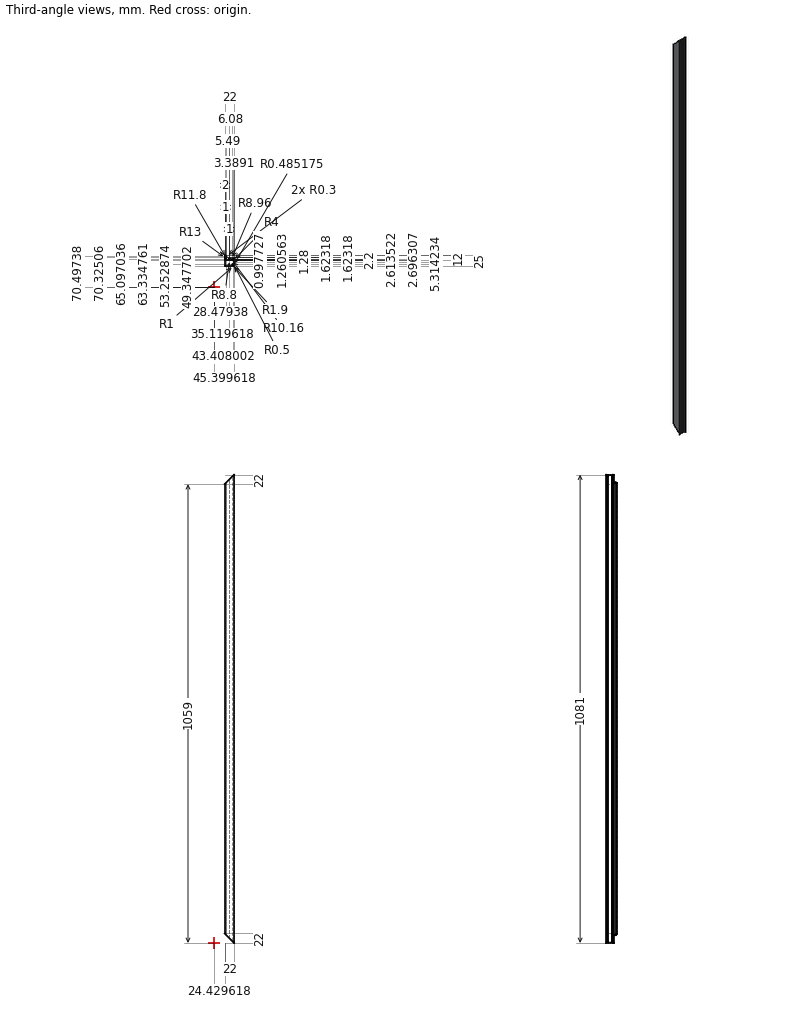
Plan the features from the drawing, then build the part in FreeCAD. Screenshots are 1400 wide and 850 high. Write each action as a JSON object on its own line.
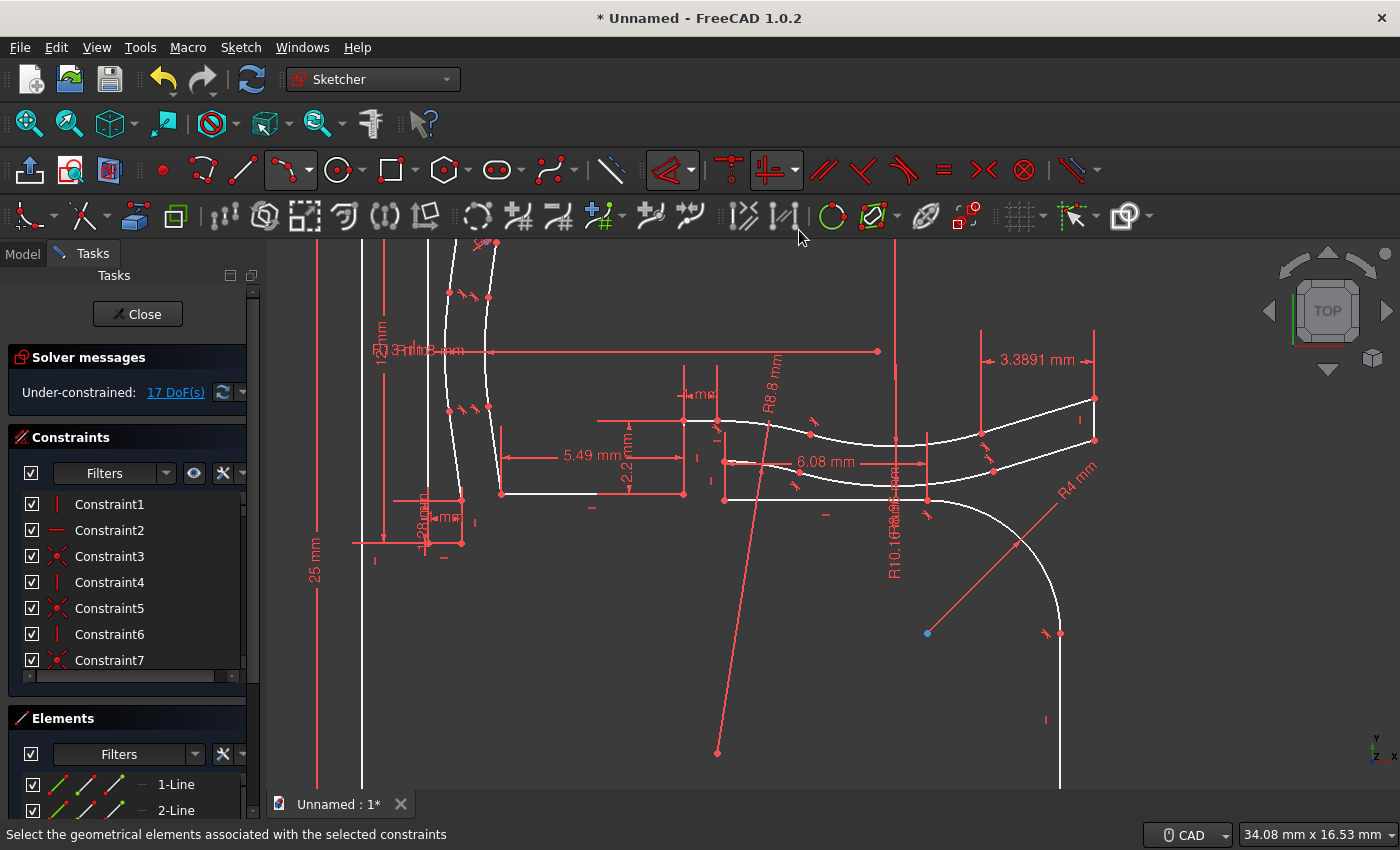
{"action": "left_click", "coordinate": [1060, 753]}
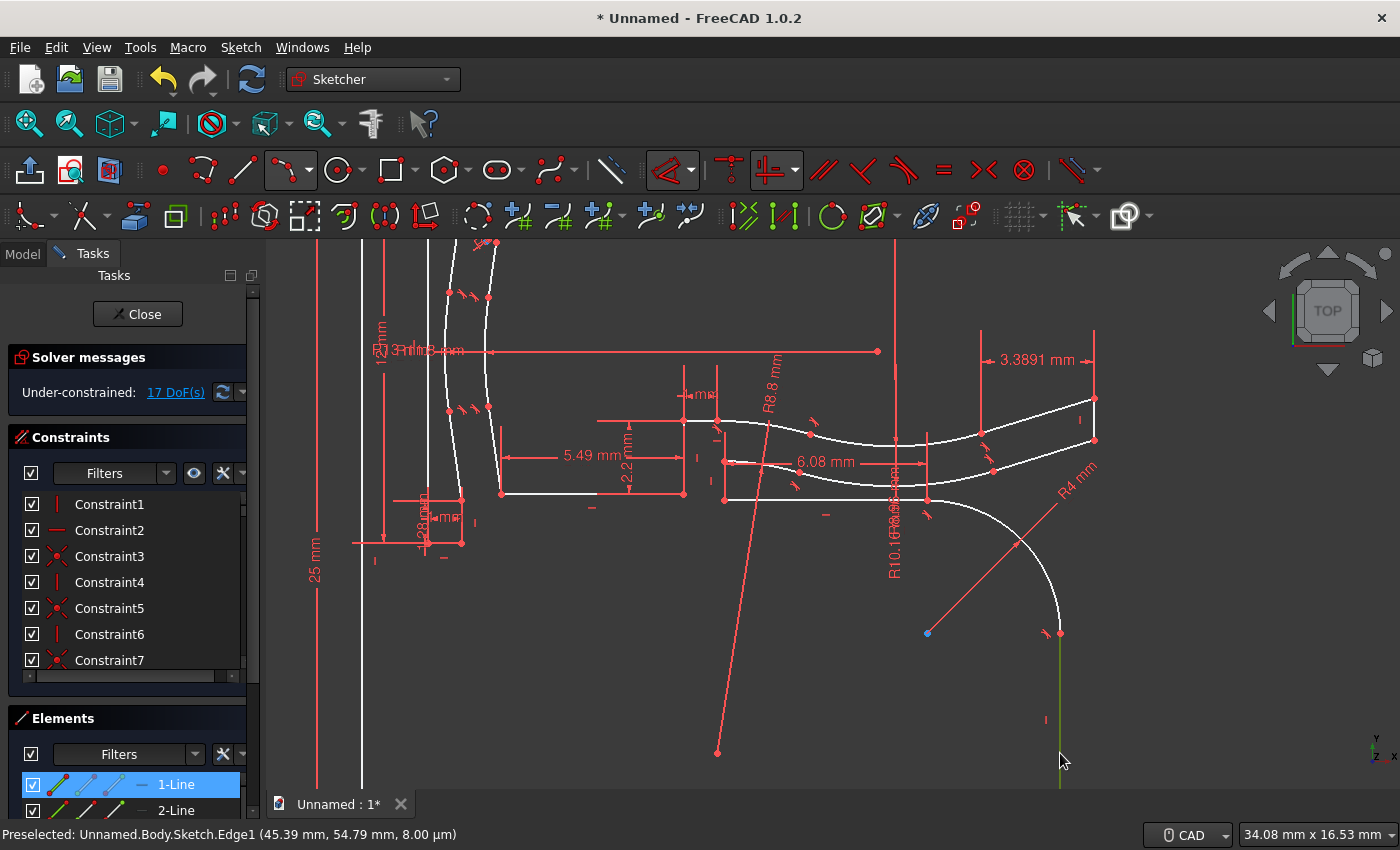
{"action": "left_click", "coordinate": [694, 170]}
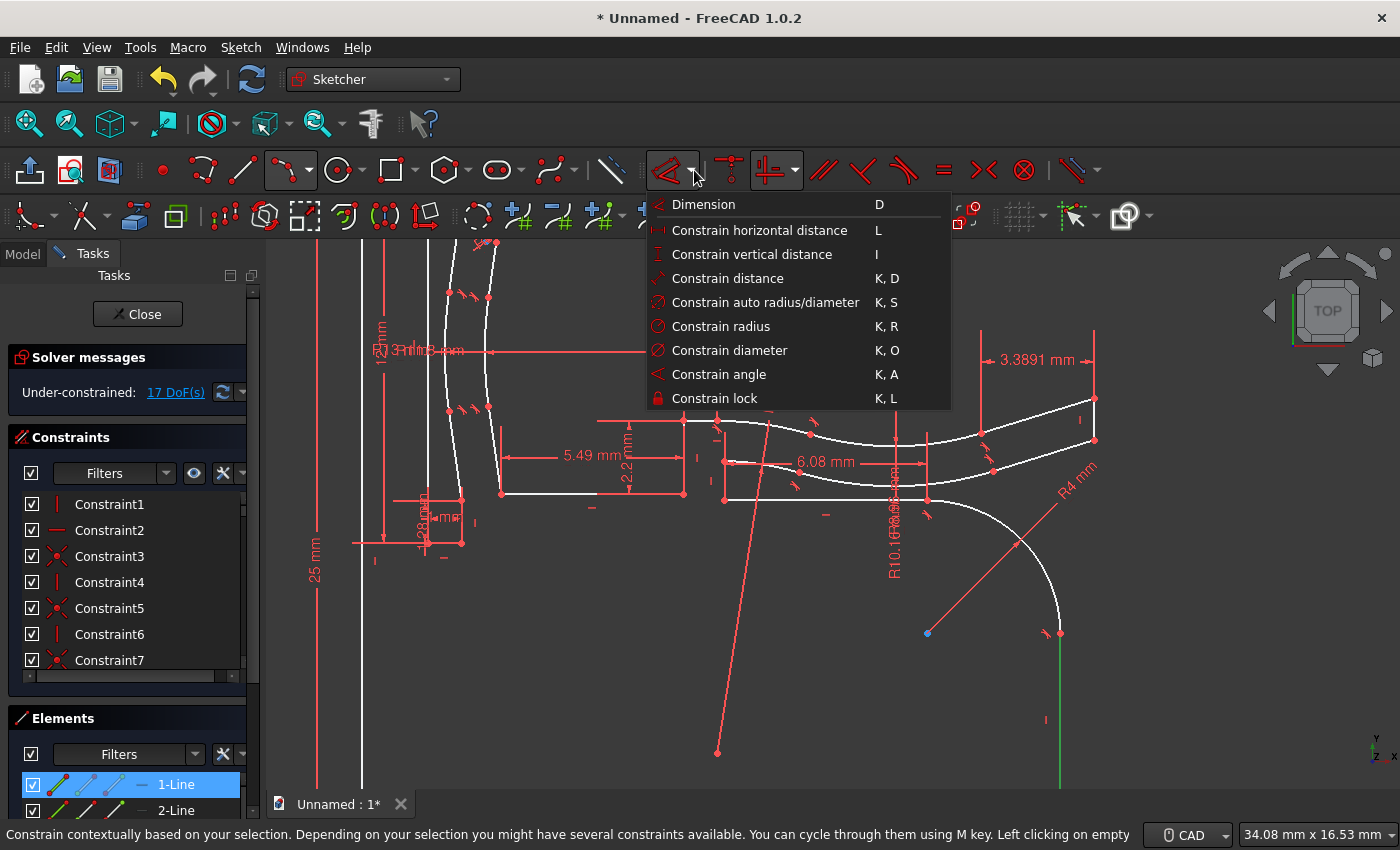
{"action": "left_click", "coordinate": [799, 254]}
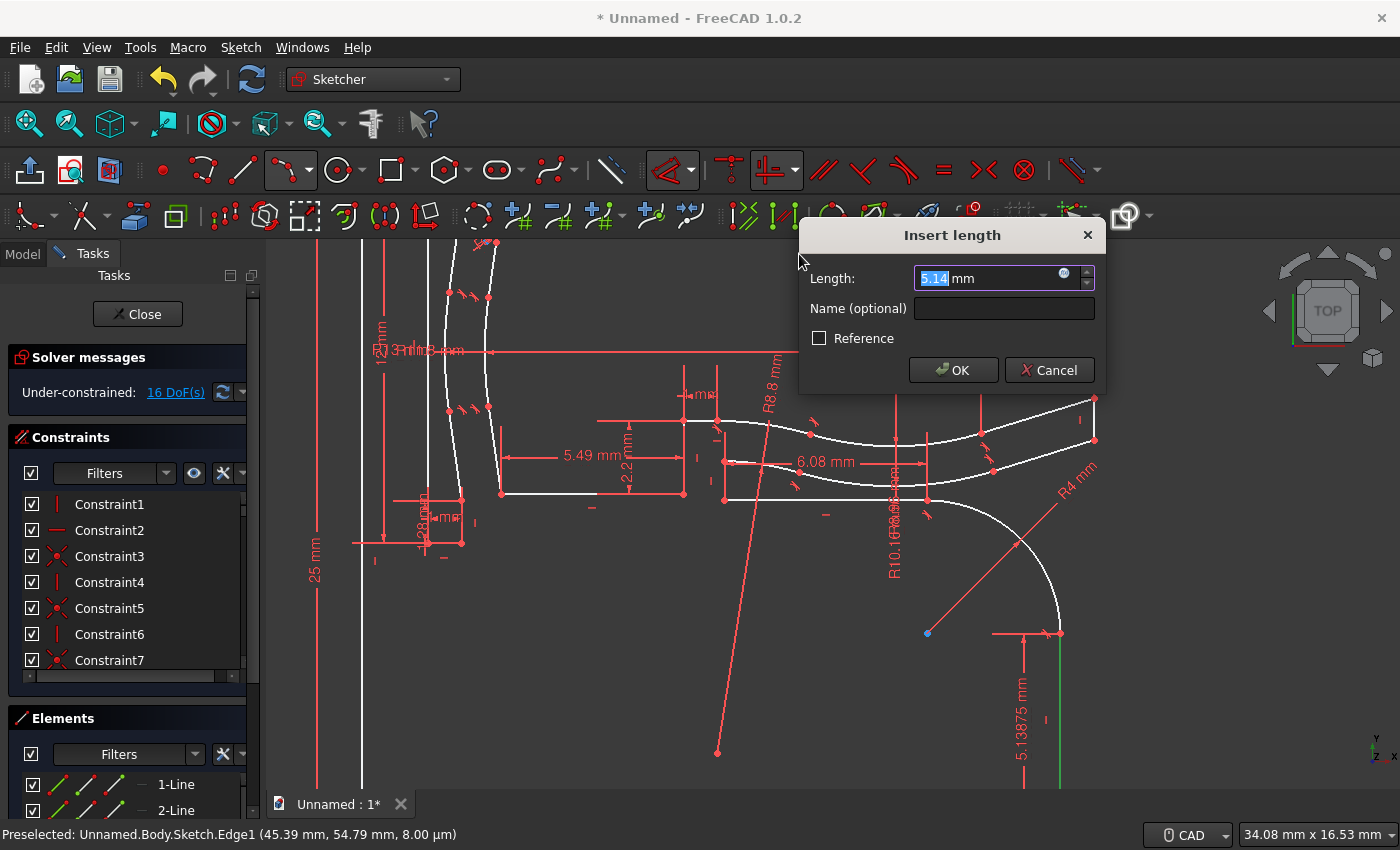
{"action": "type", "text": "5.314234"}
{"action": "key", "text": "Return"}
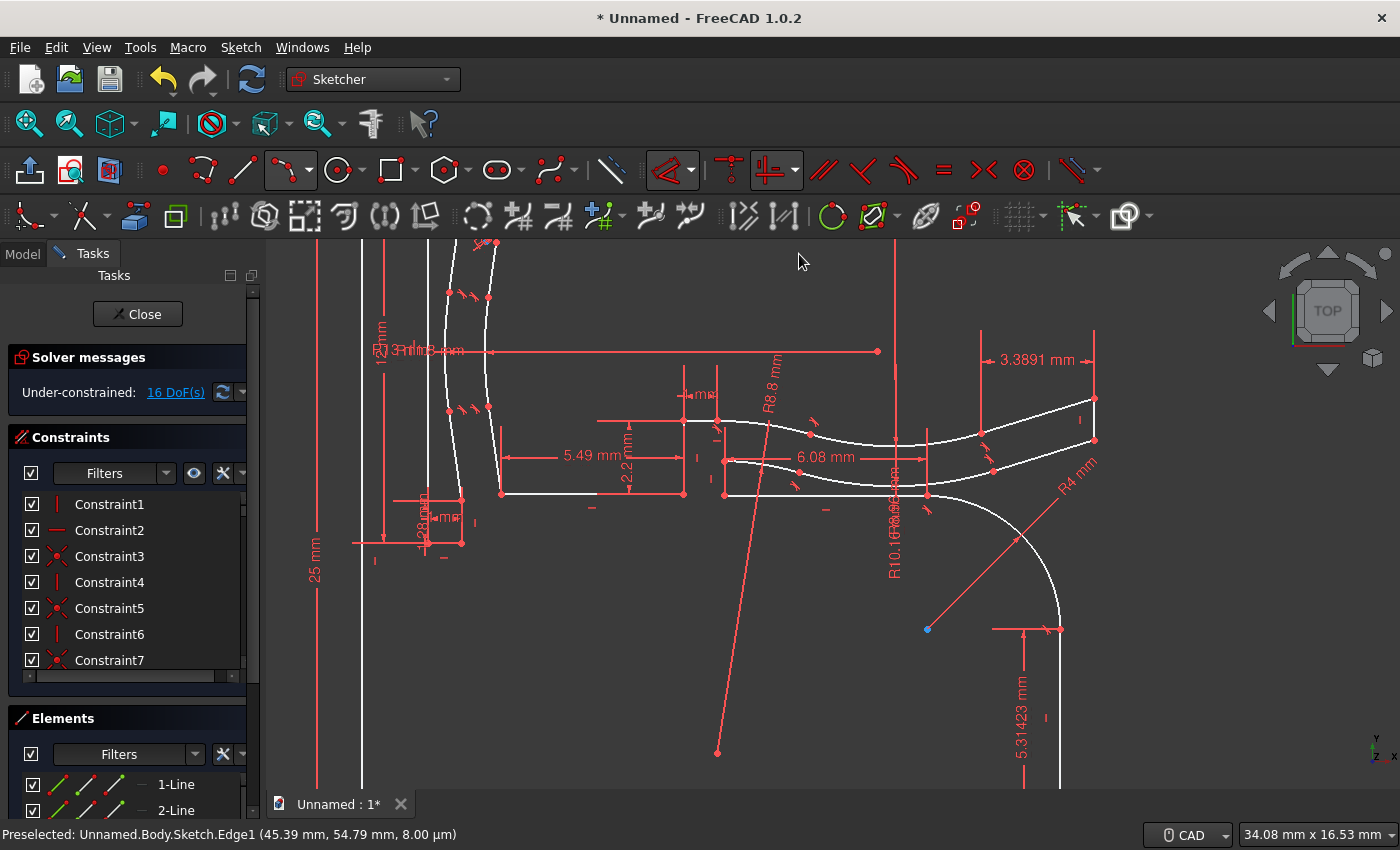
{"action": "scroll", "coordinate": [725, 485], "scroll_direction": "up", "scroll_amount": 2}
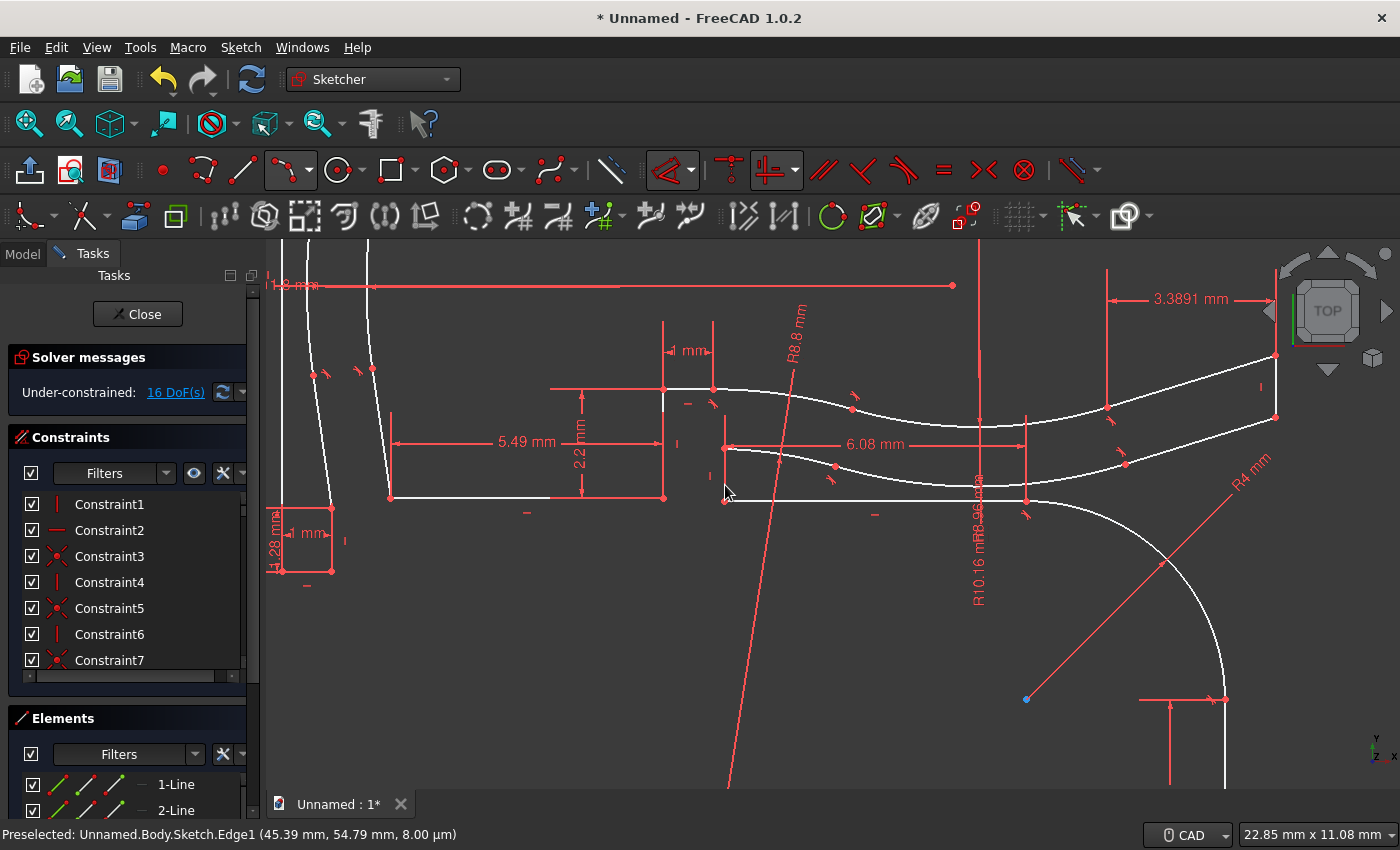
{"action": "left_click", "coordinate": [725, 485]}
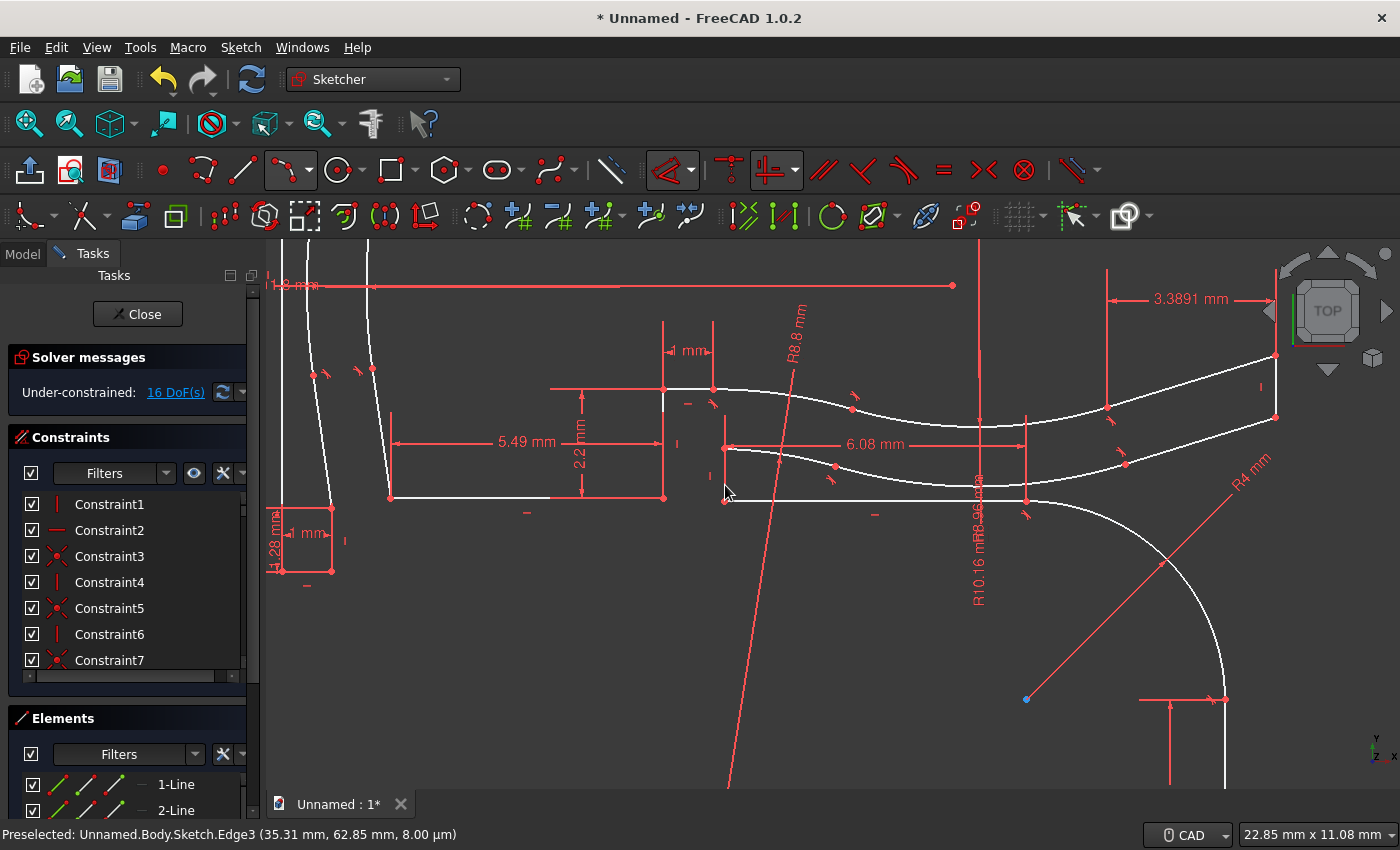
{"action": "left_click", "coordinate": [694, 170]}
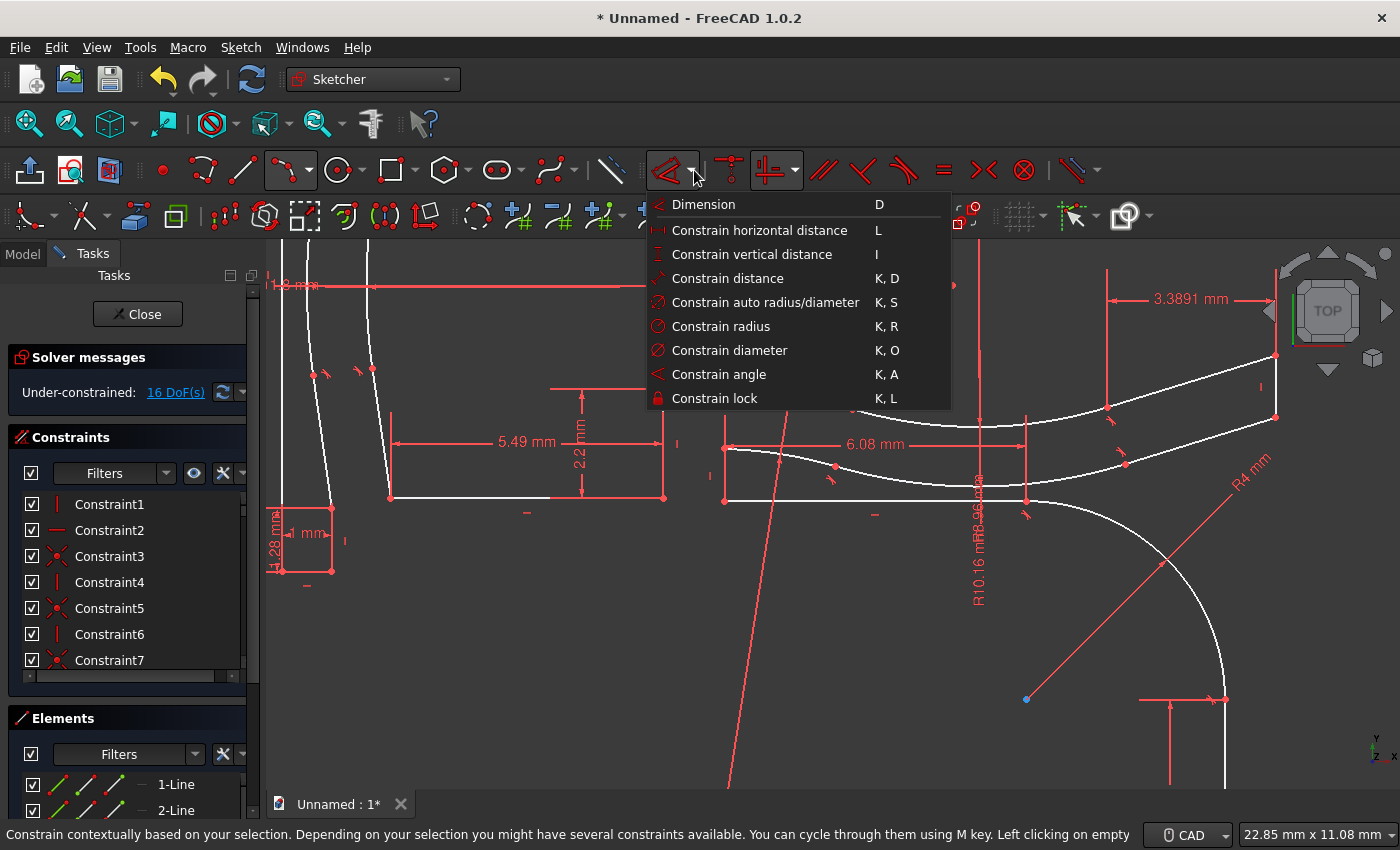
{"action": "left_click", "coordinate": [799, 254]}